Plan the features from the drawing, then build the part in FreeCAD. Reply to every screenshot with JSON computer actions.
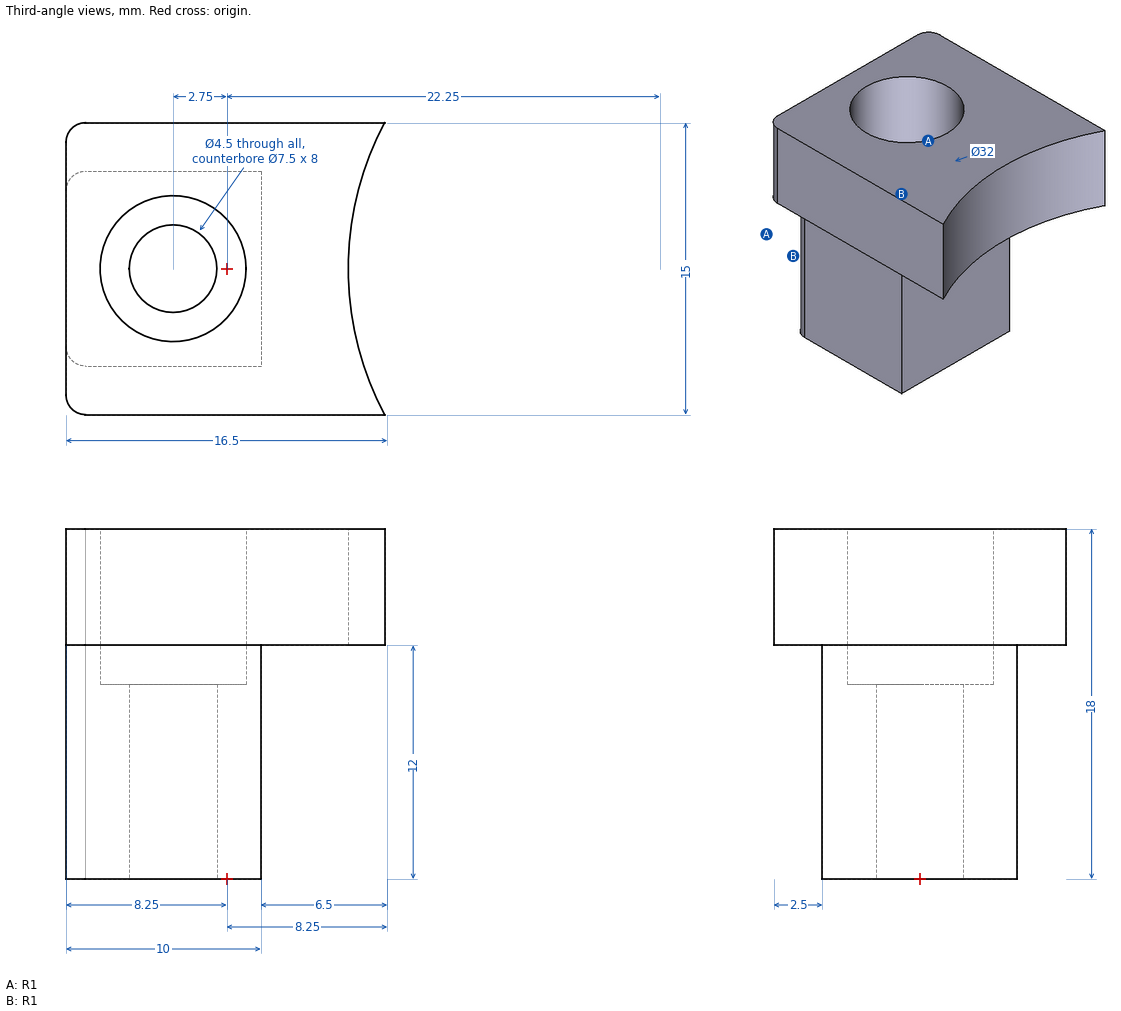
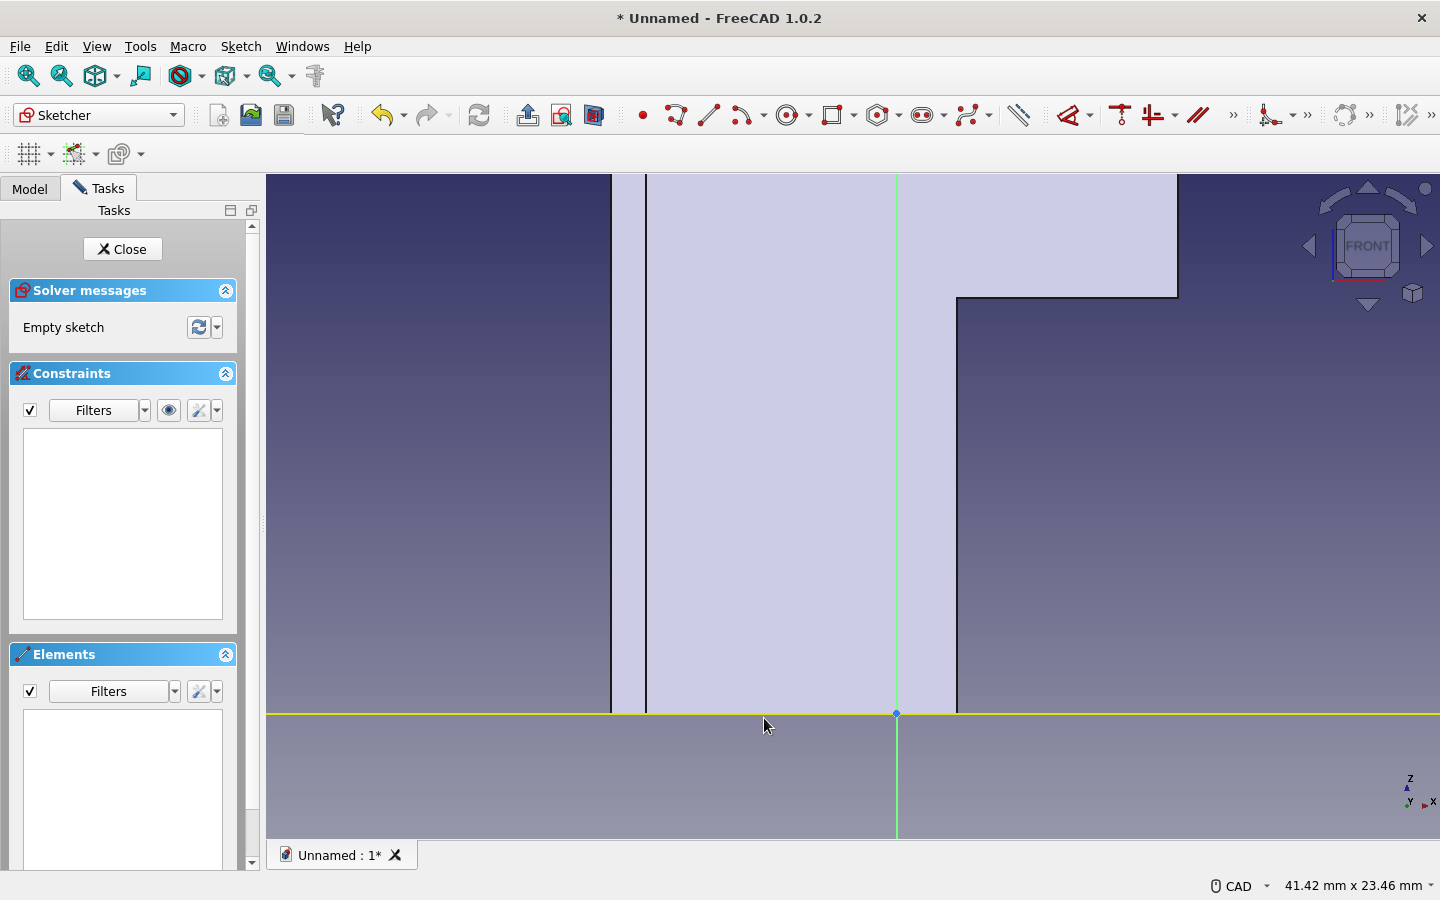
{"action": "key", "text": "g r"}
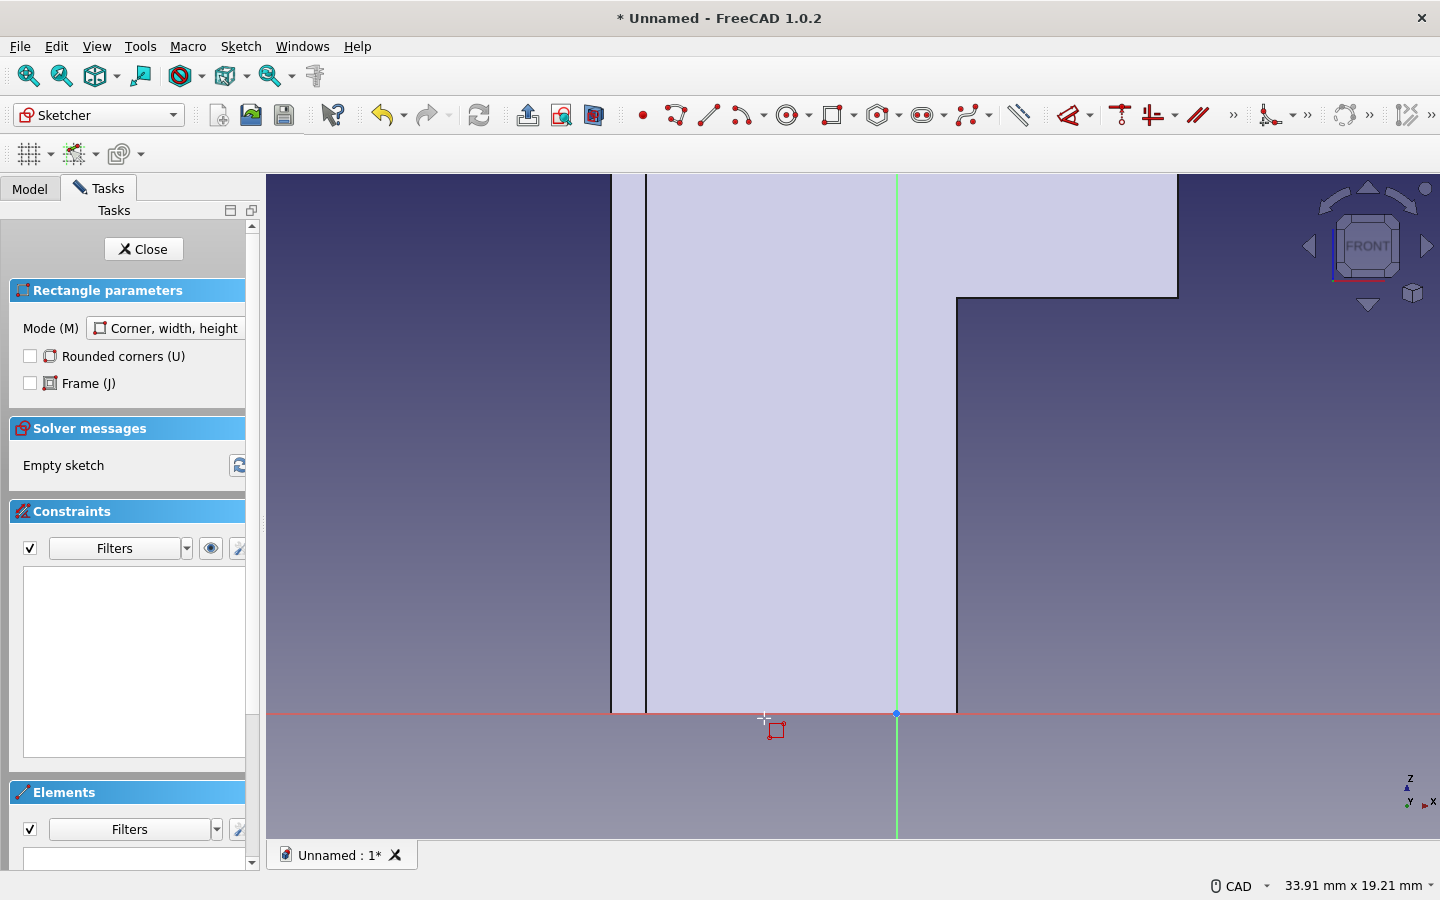
{"action": "left_click", "coordinate": [611, 298]}
{"action": "left_click", "coordinate": [957, 714]}
{"action": "key", "text": "Escape"}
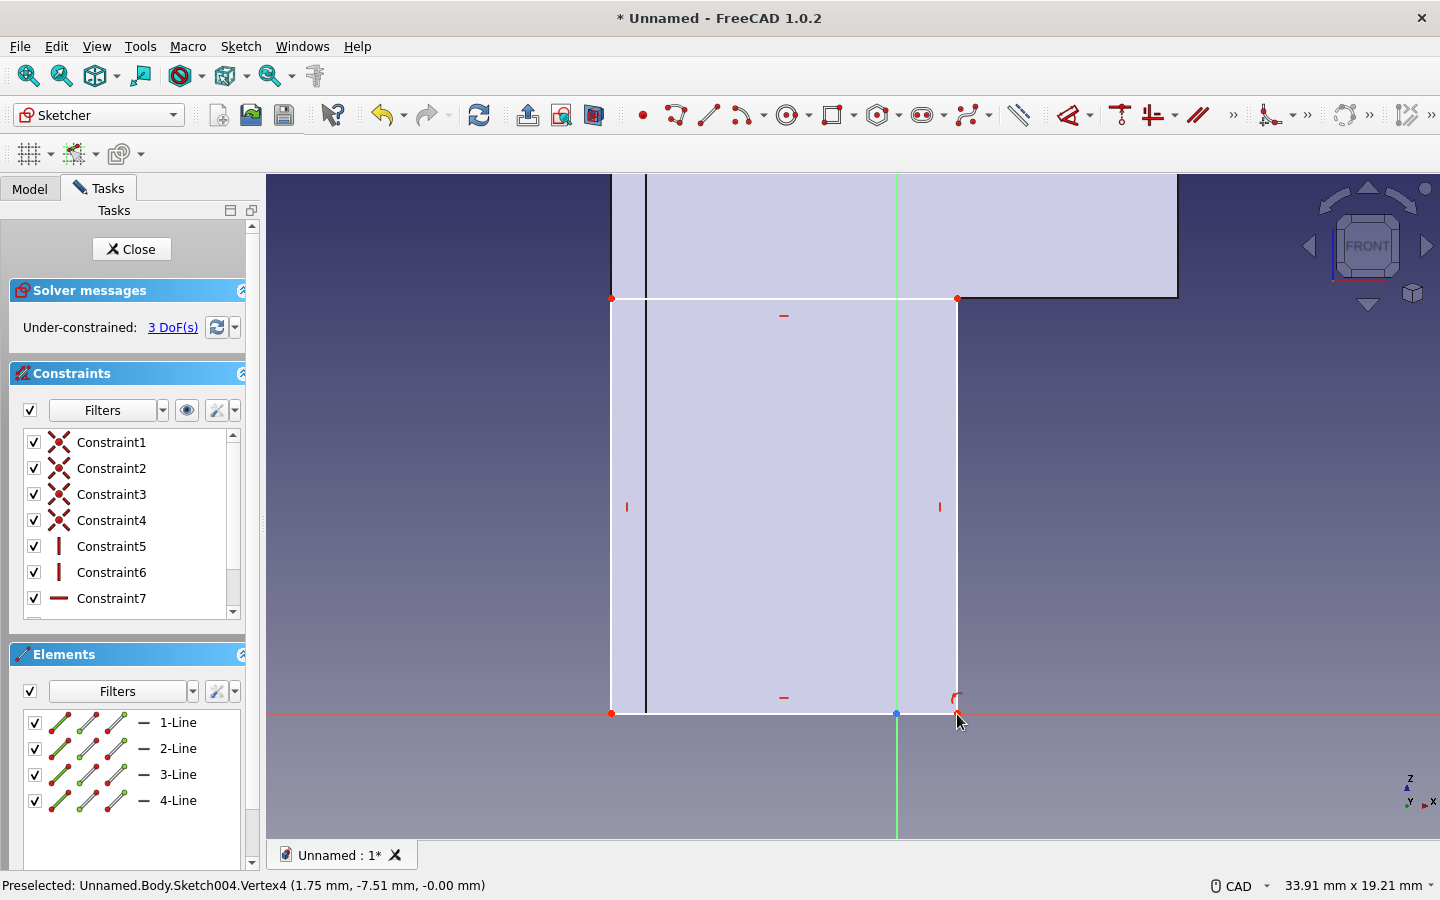
{"action": "key", "text": "d"}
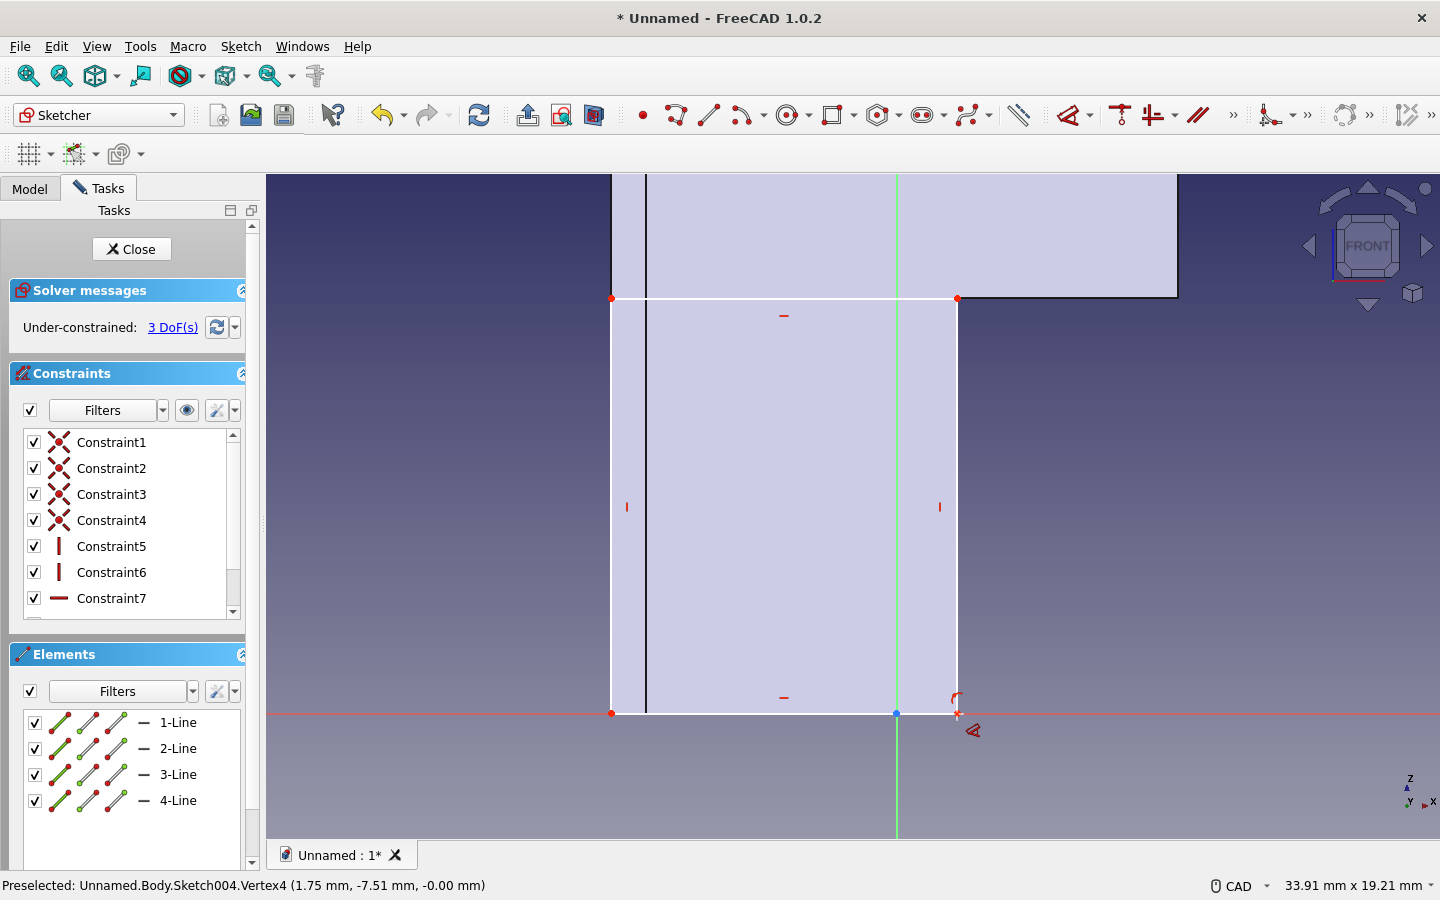
{"action": "left_click", "coordinate": [611, 423]}
{"action": "left_click", "coordinate": [577, 506]}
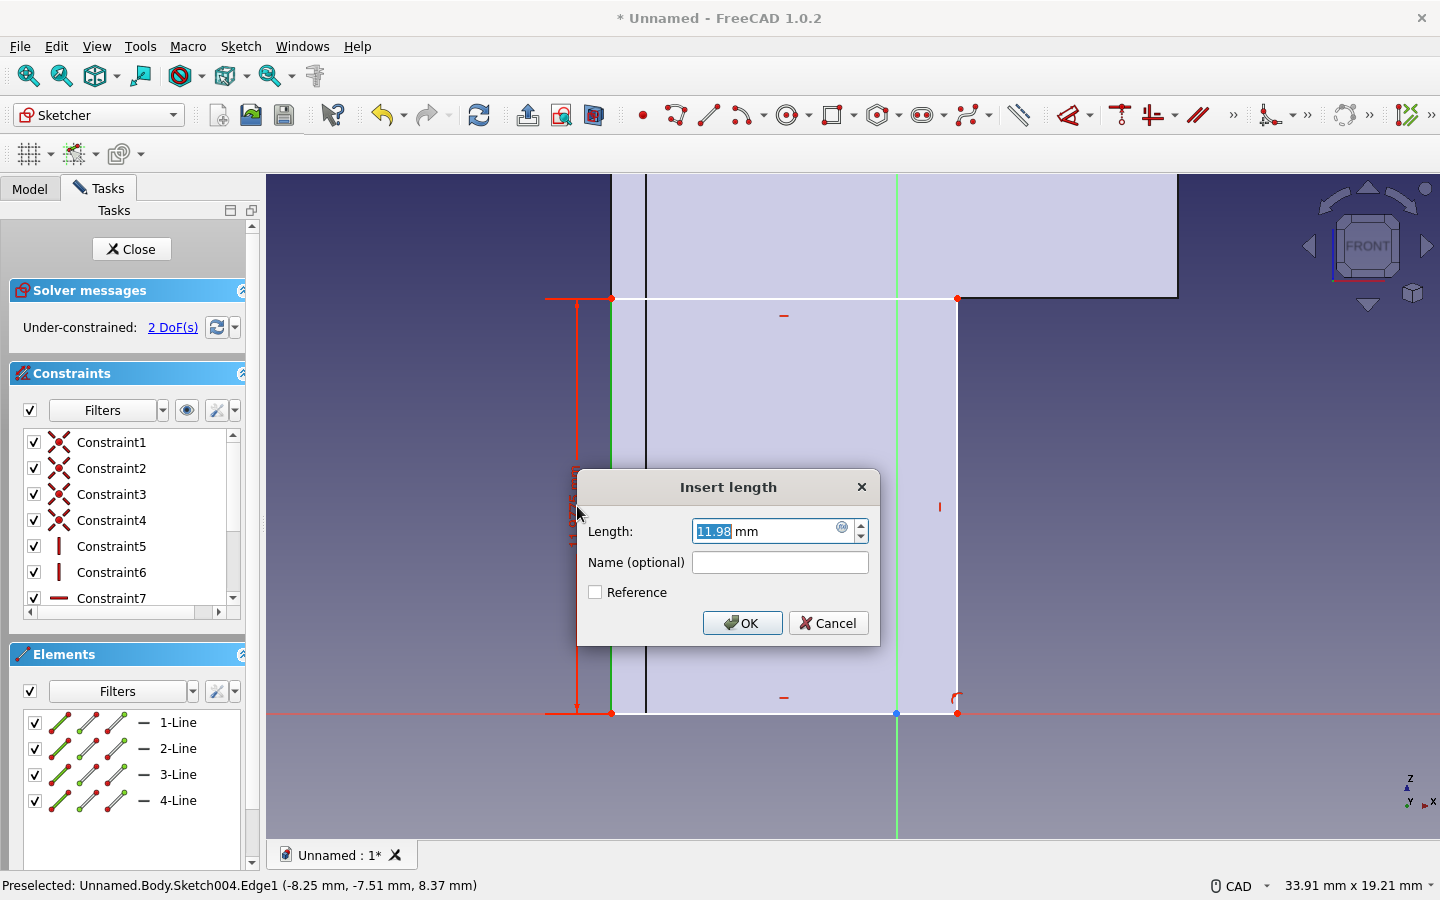
{"action": "type", "text": "12"}
{"action": "key", "text": "Return"}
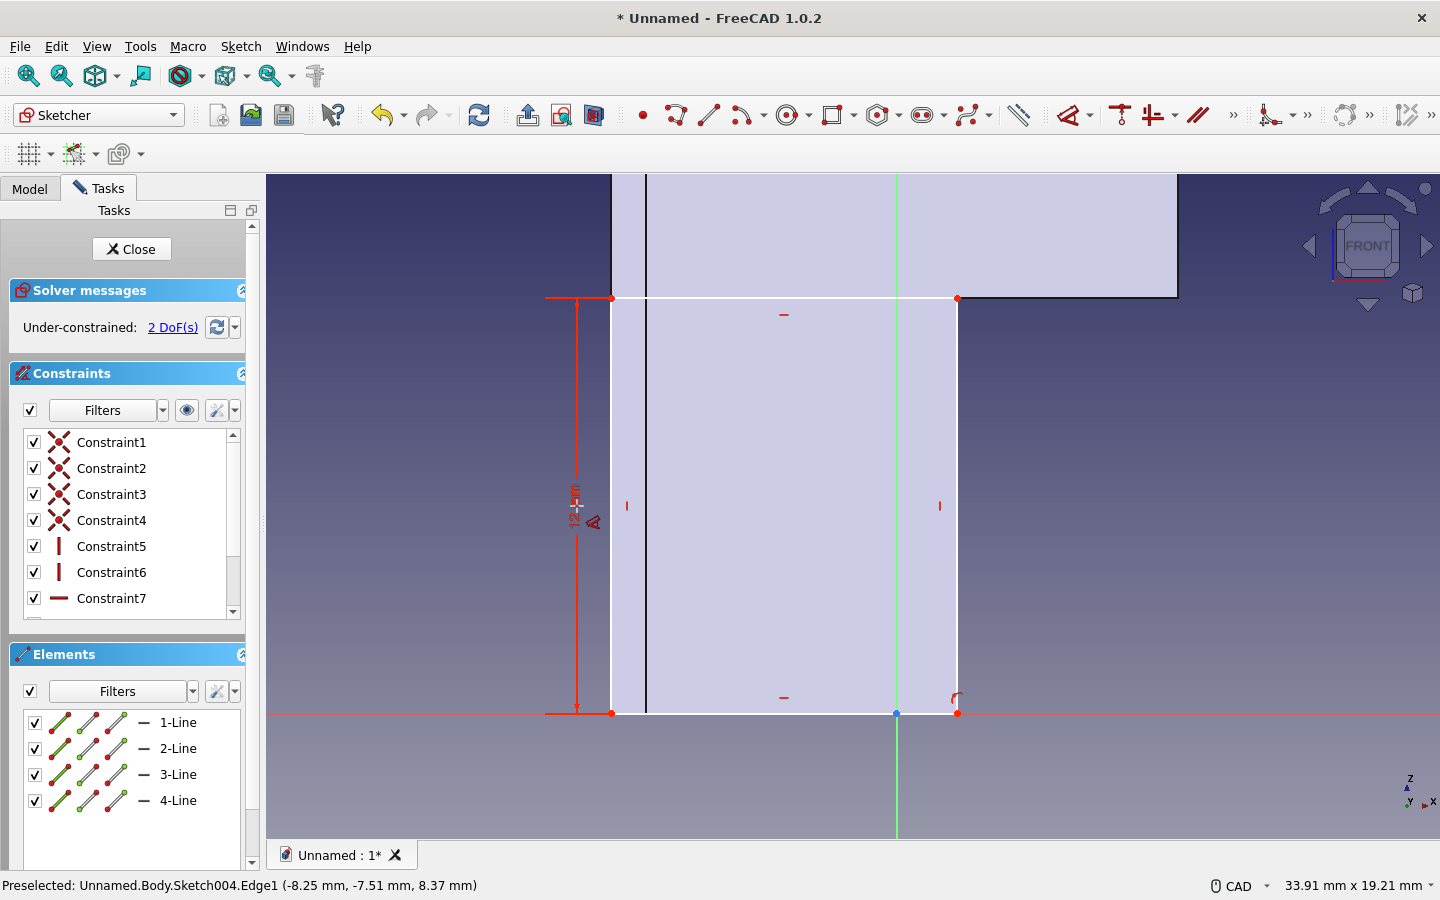
{"action": "left_click", "coordinate": [715, 714]}
{"action": "left_click", "coordinate": [784, 748]}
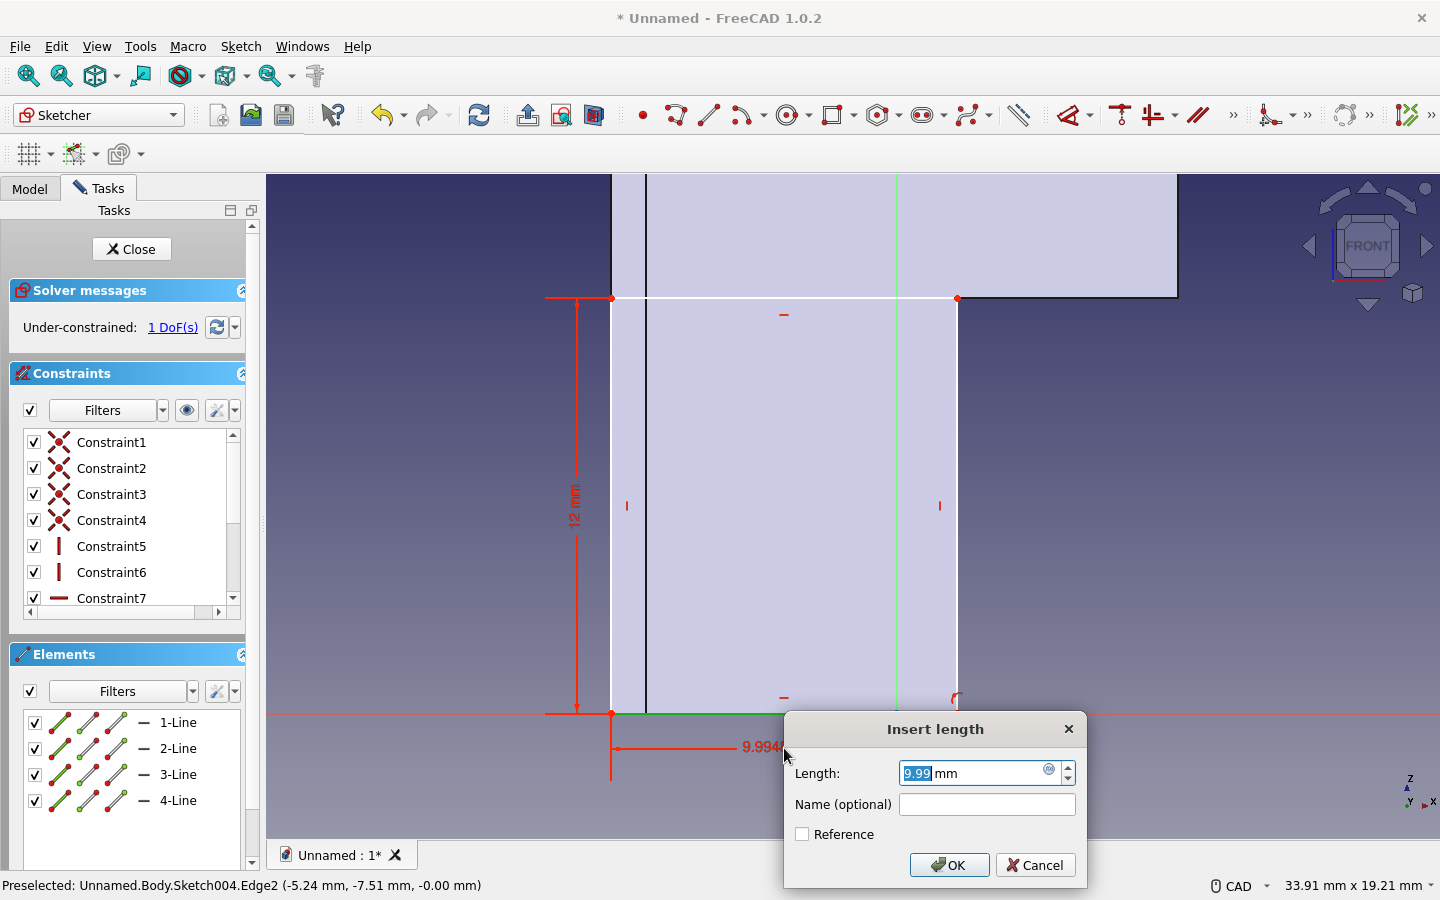
{"action": "type", "text": "10"}
{"action": "key", "text": "Return"}